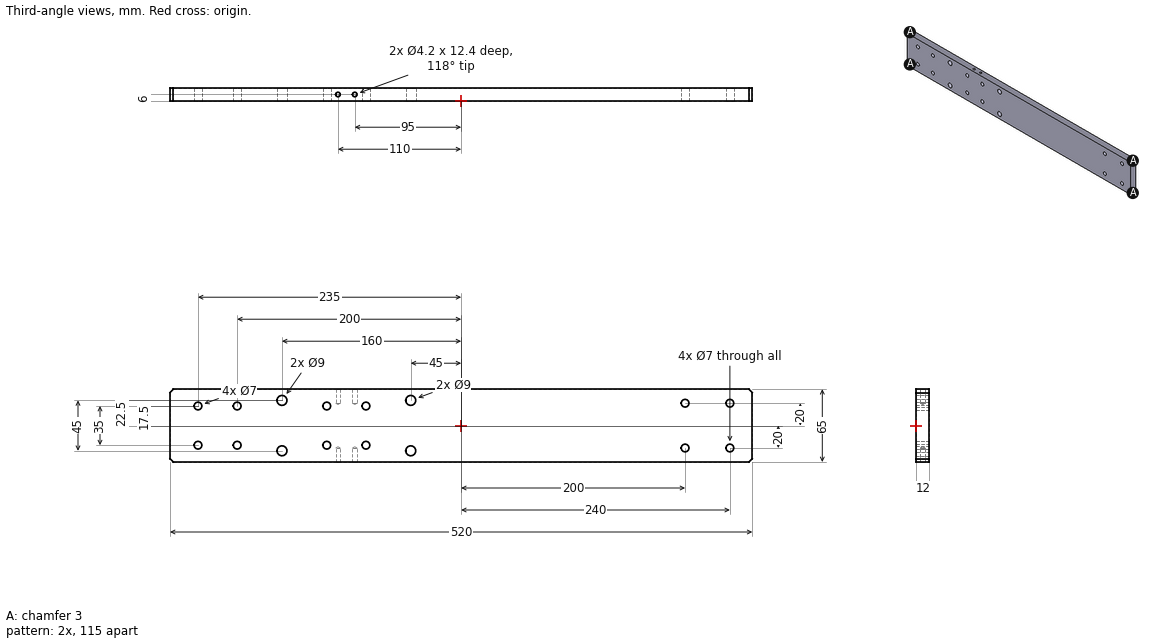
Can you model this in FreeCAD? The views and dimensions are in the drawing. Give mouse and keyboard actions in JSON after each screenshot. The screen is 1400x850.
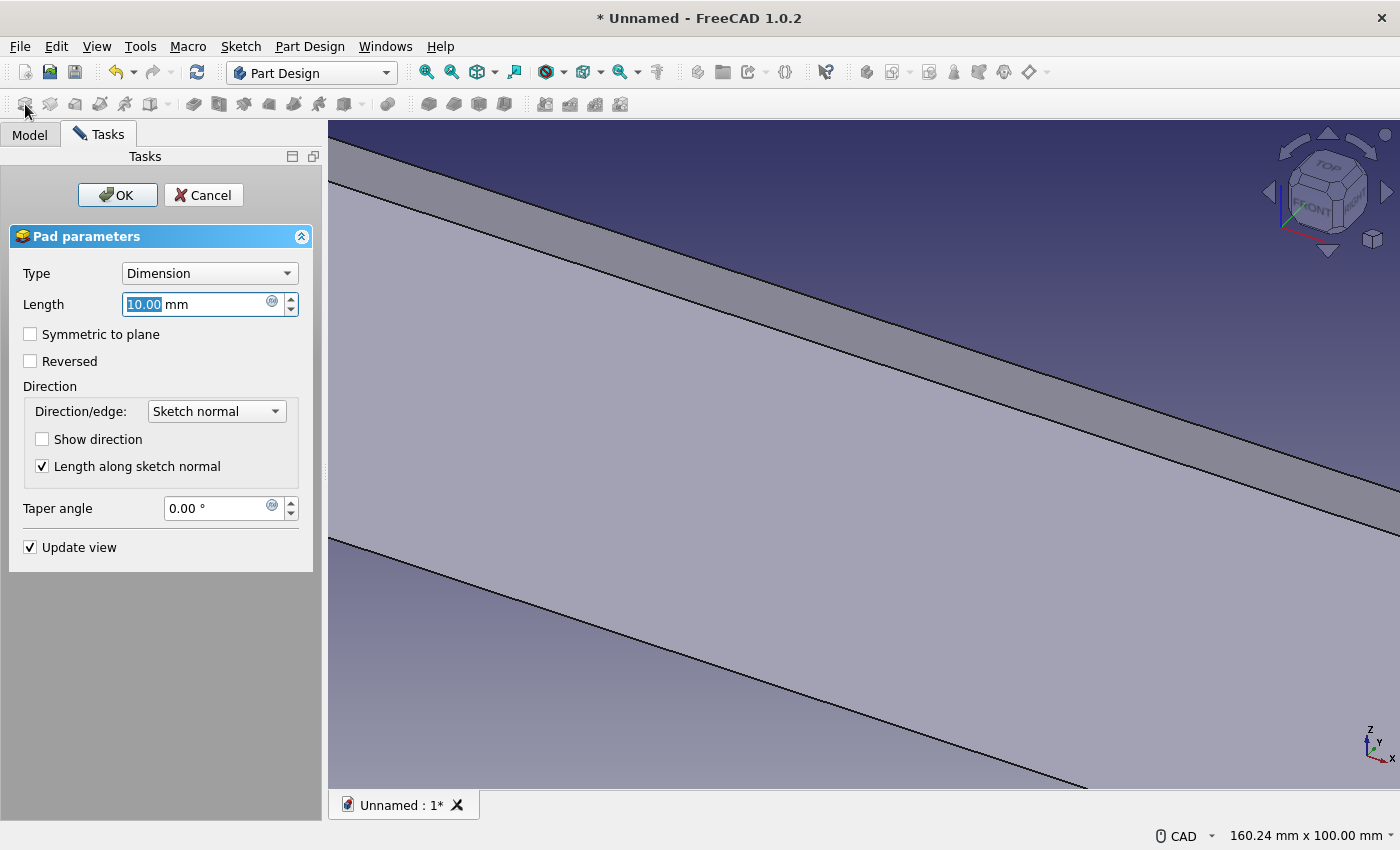
{"action": "type", "text": "12"}
{"action": "key", "text": "Tab"}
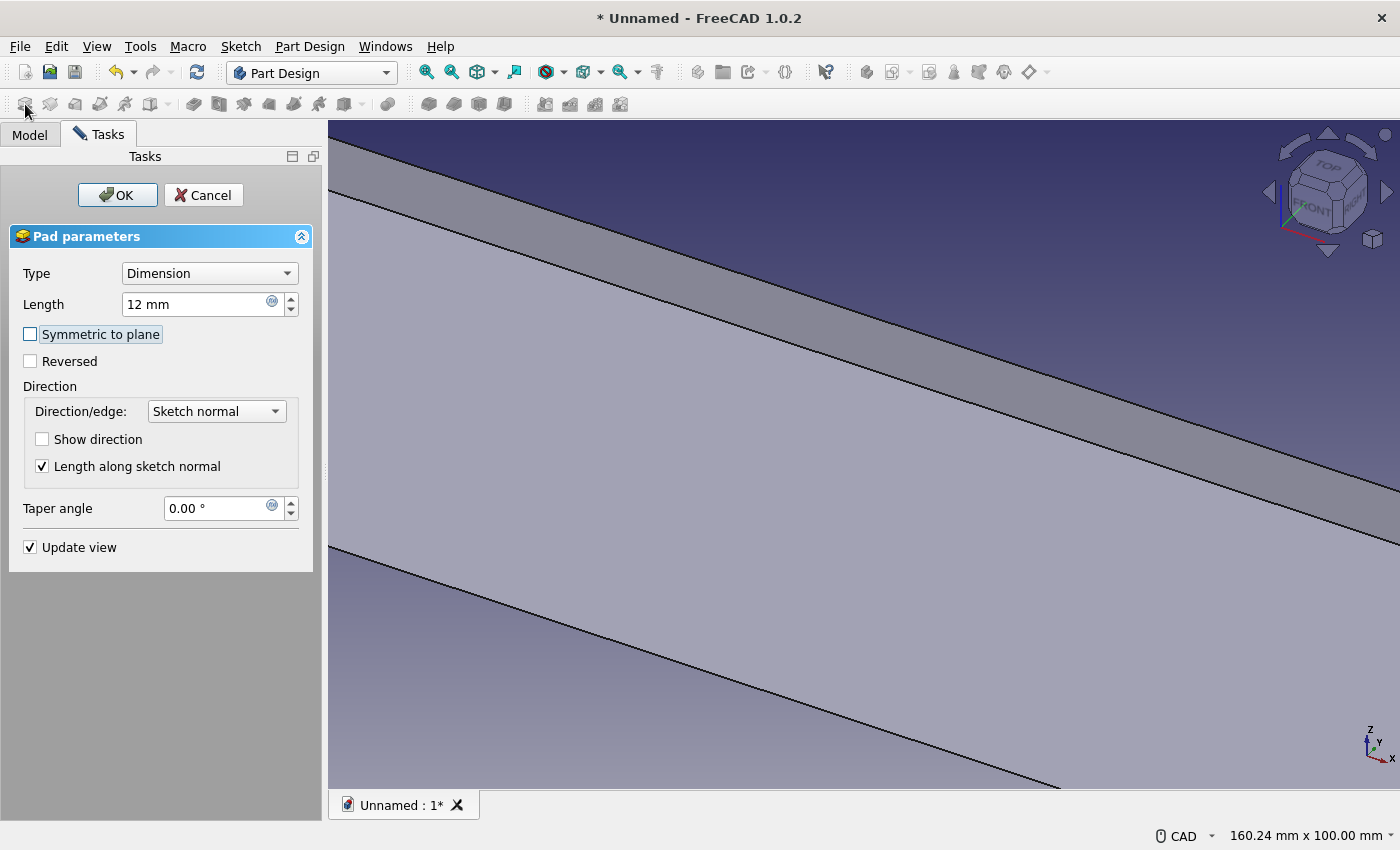
{"action": "left_click", "coordinate": [31, 361]}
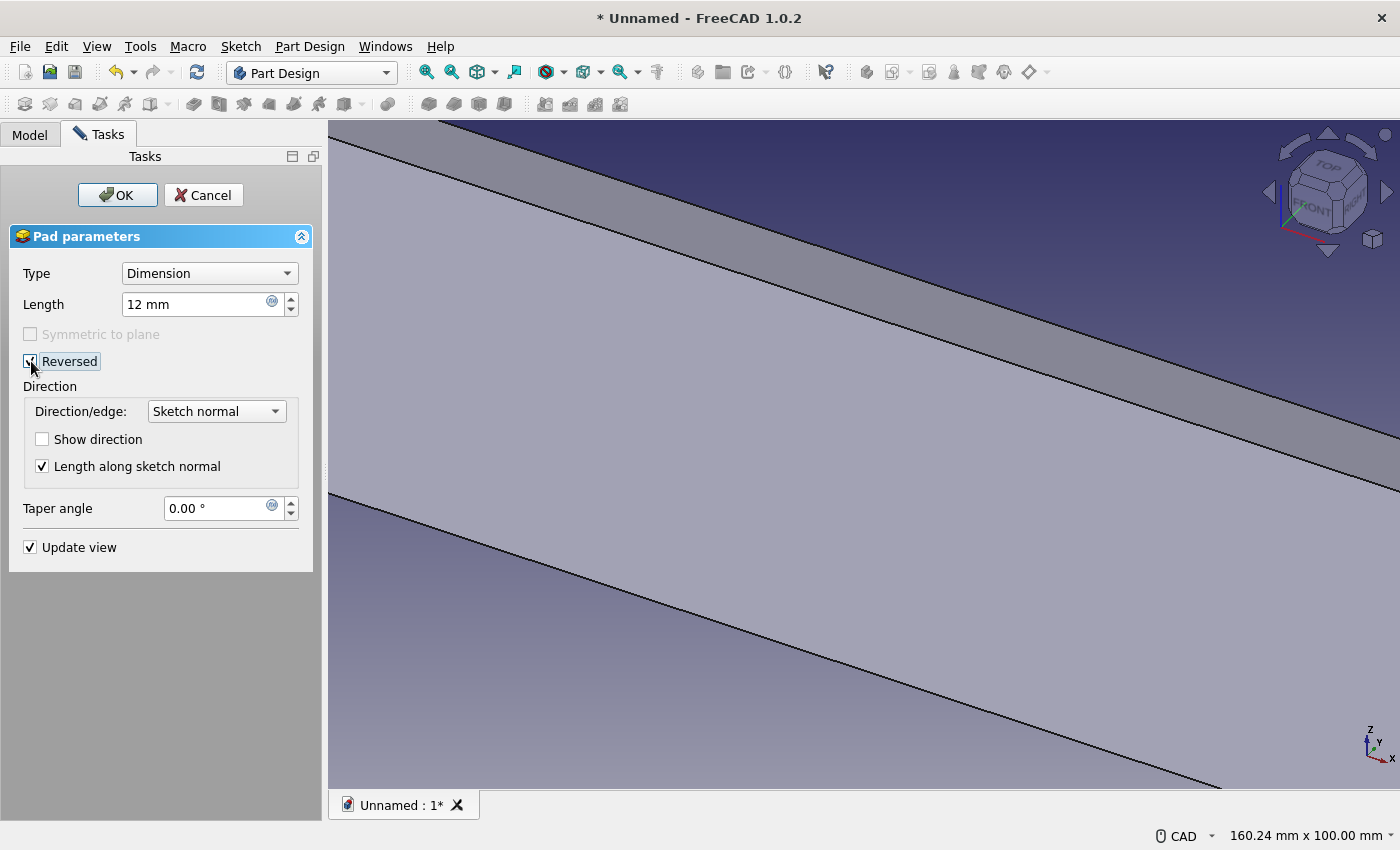
{"action": "left_click", "coordinate": [118, 195]}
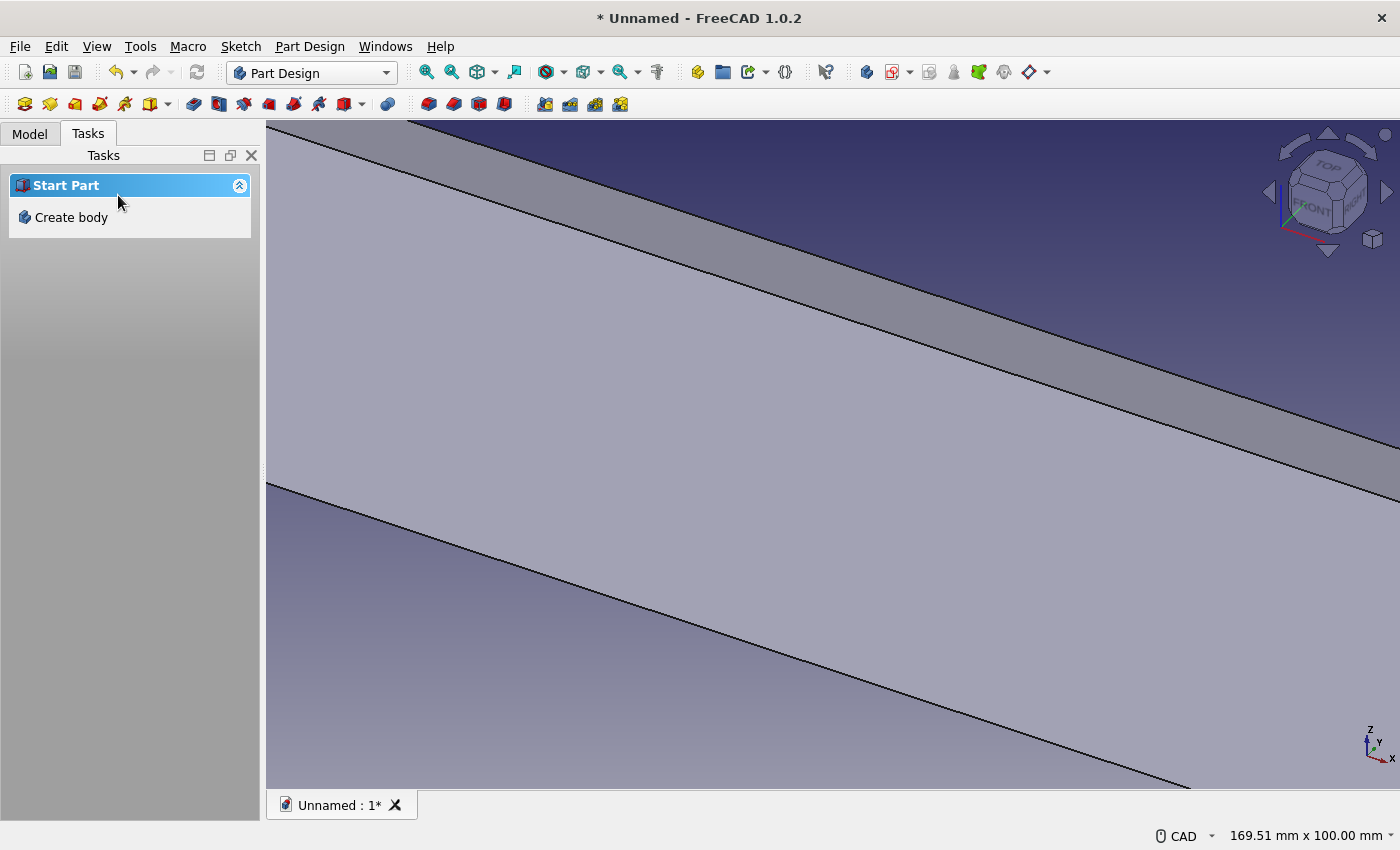
{"action": "left_click", "coordinate": [427, 72]}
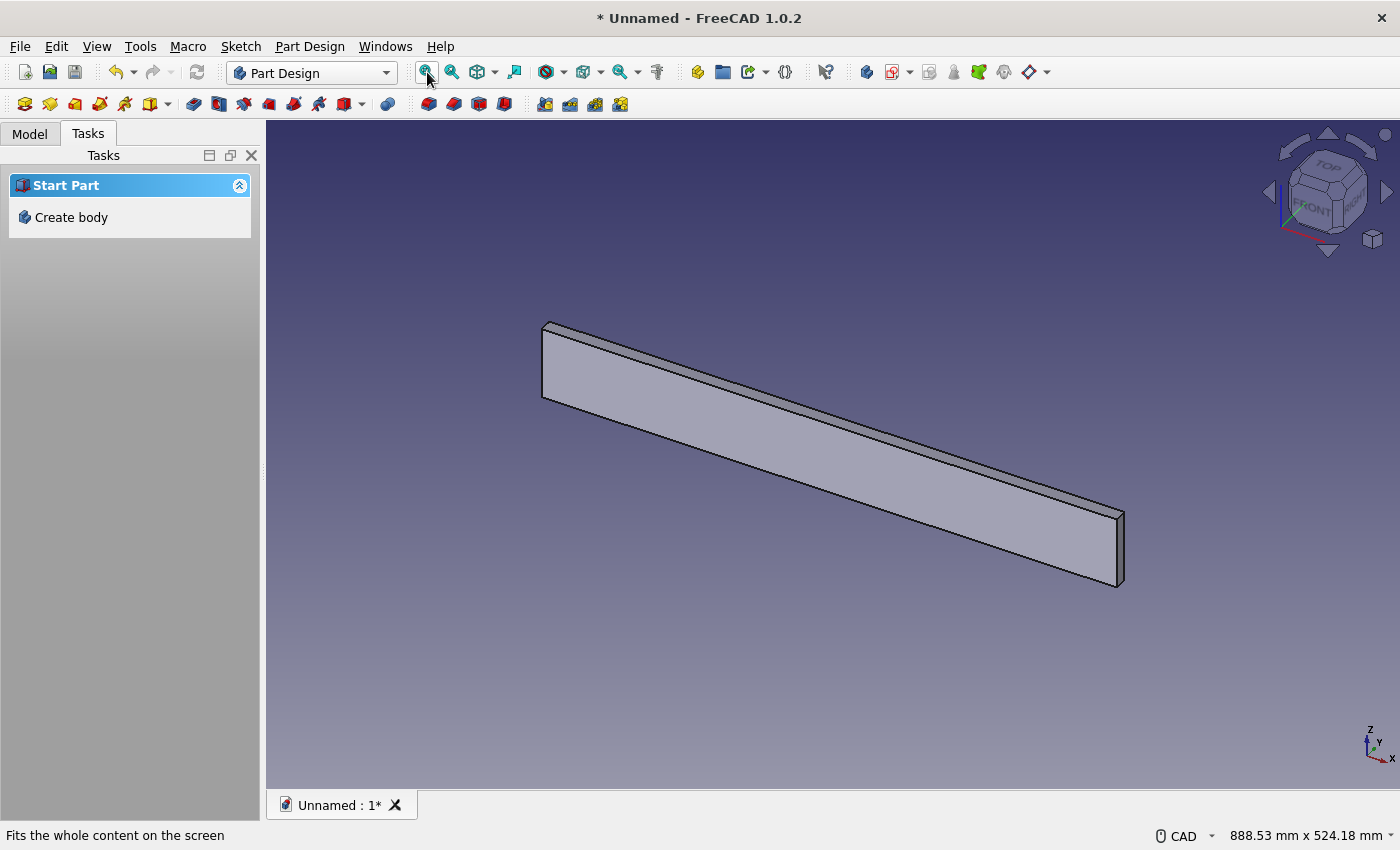
{"action": "left_click", "coordinate": [1075, 539]}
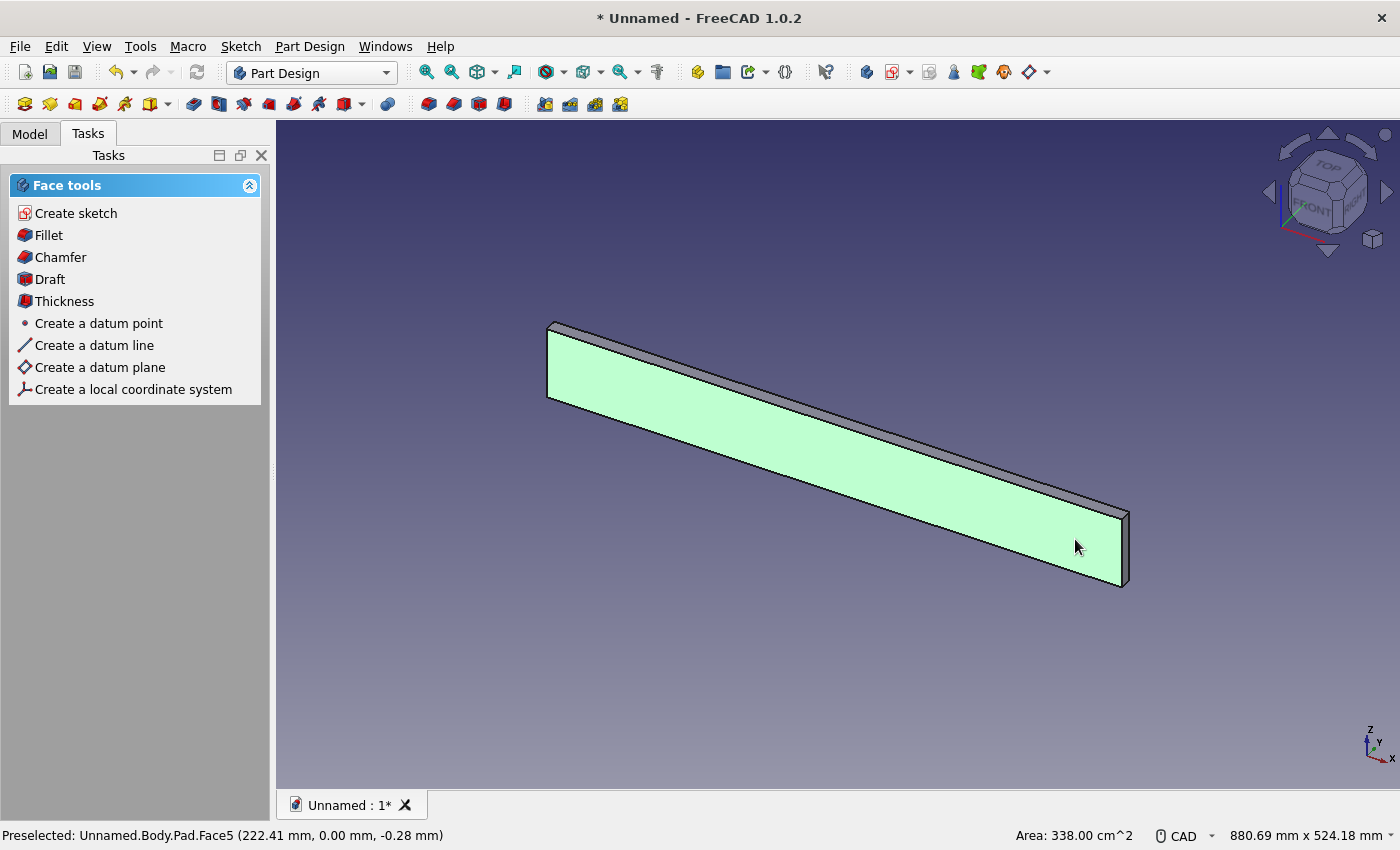
{"action": "left_click", "coordinate": [892, 72]}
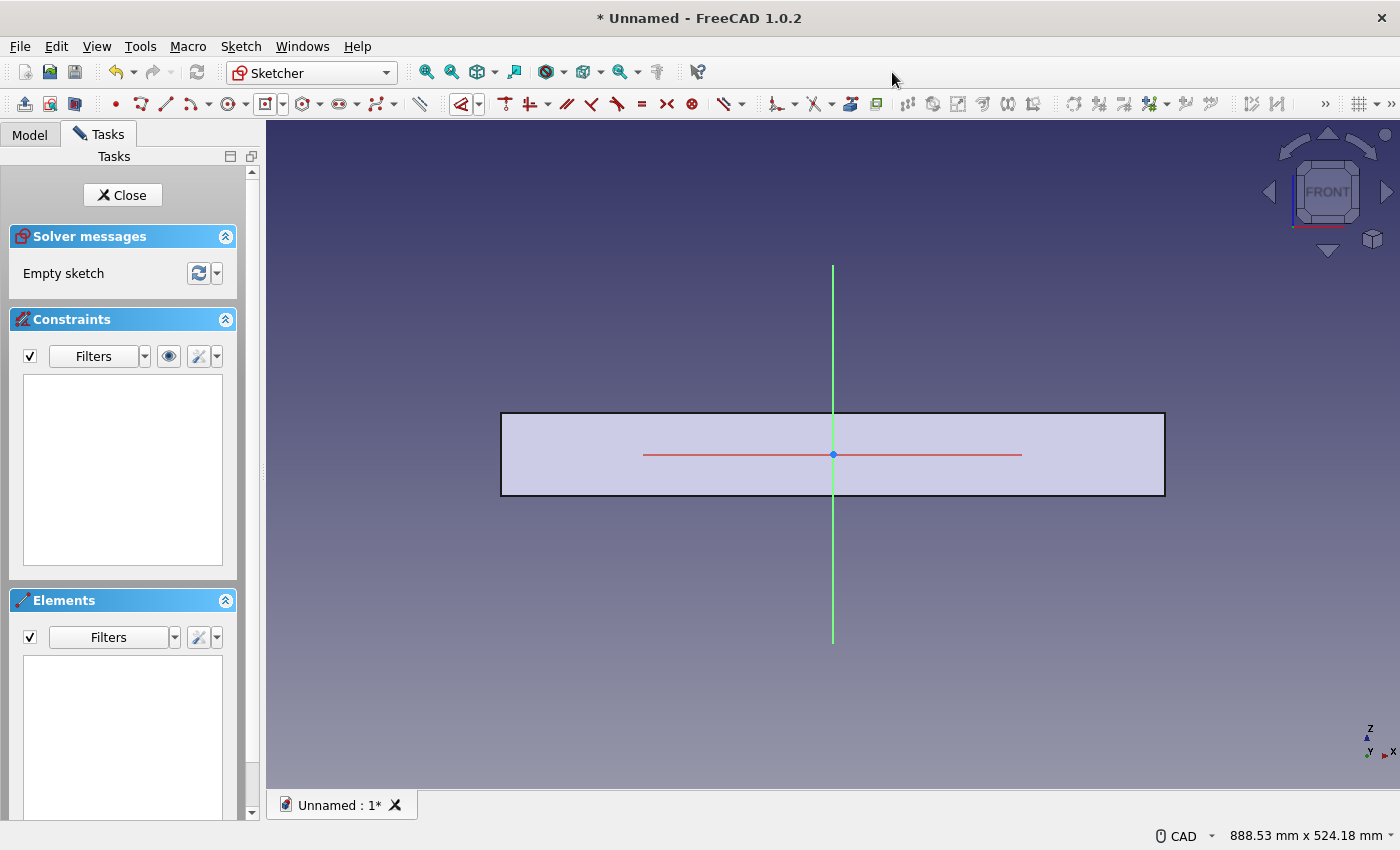
{"action": "scroll", "coordinate": [1168, 455], "scroll_direction": "up", "scroll_amount": 10}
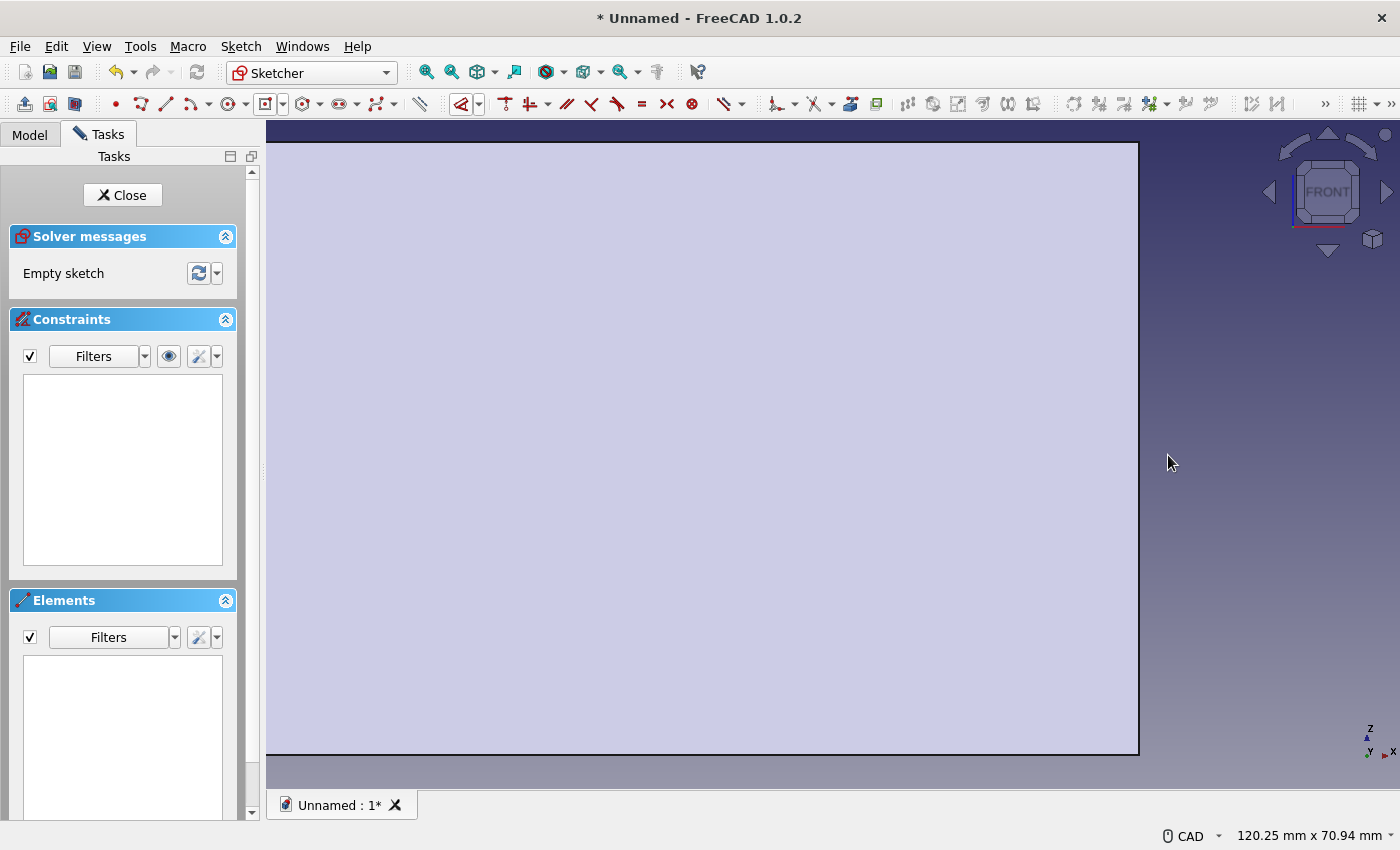
{"action": "left_click", "coordinate": [228, 104]}